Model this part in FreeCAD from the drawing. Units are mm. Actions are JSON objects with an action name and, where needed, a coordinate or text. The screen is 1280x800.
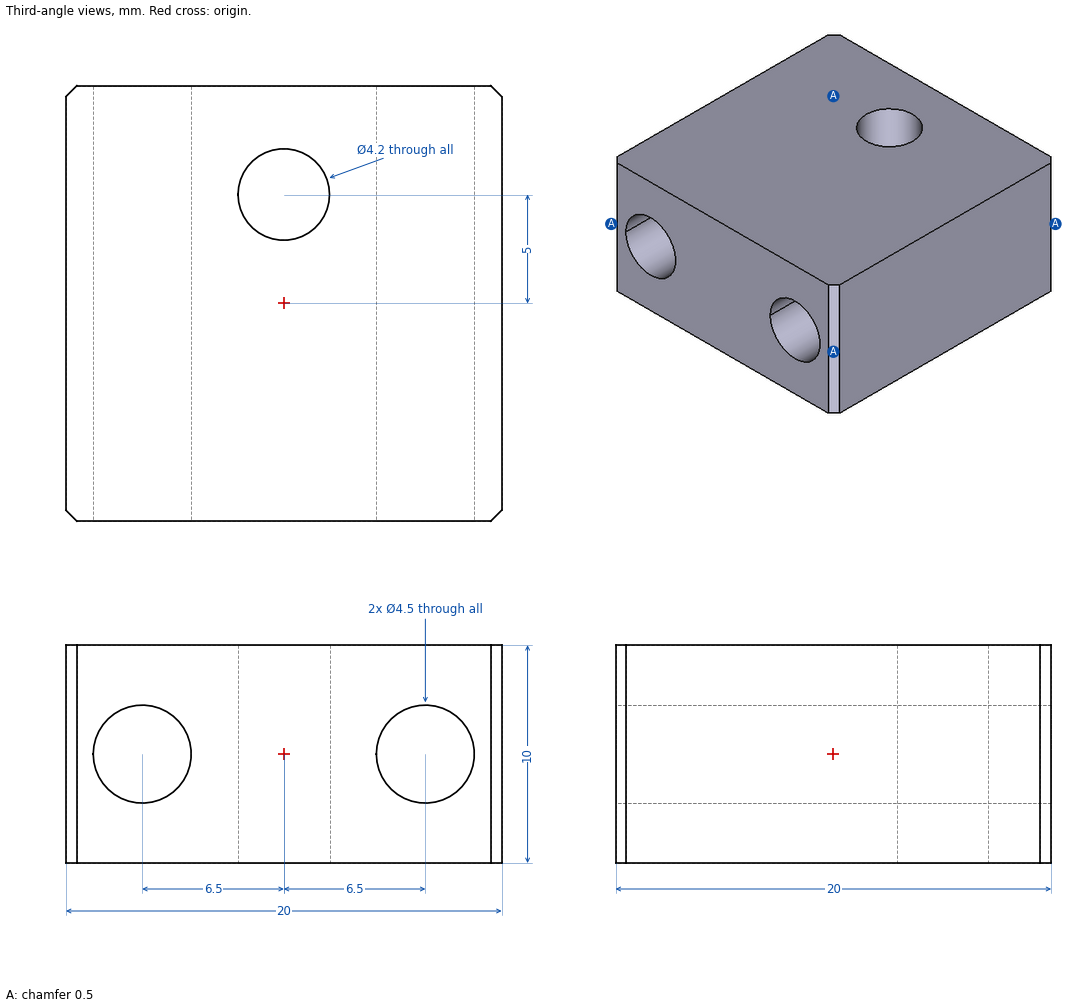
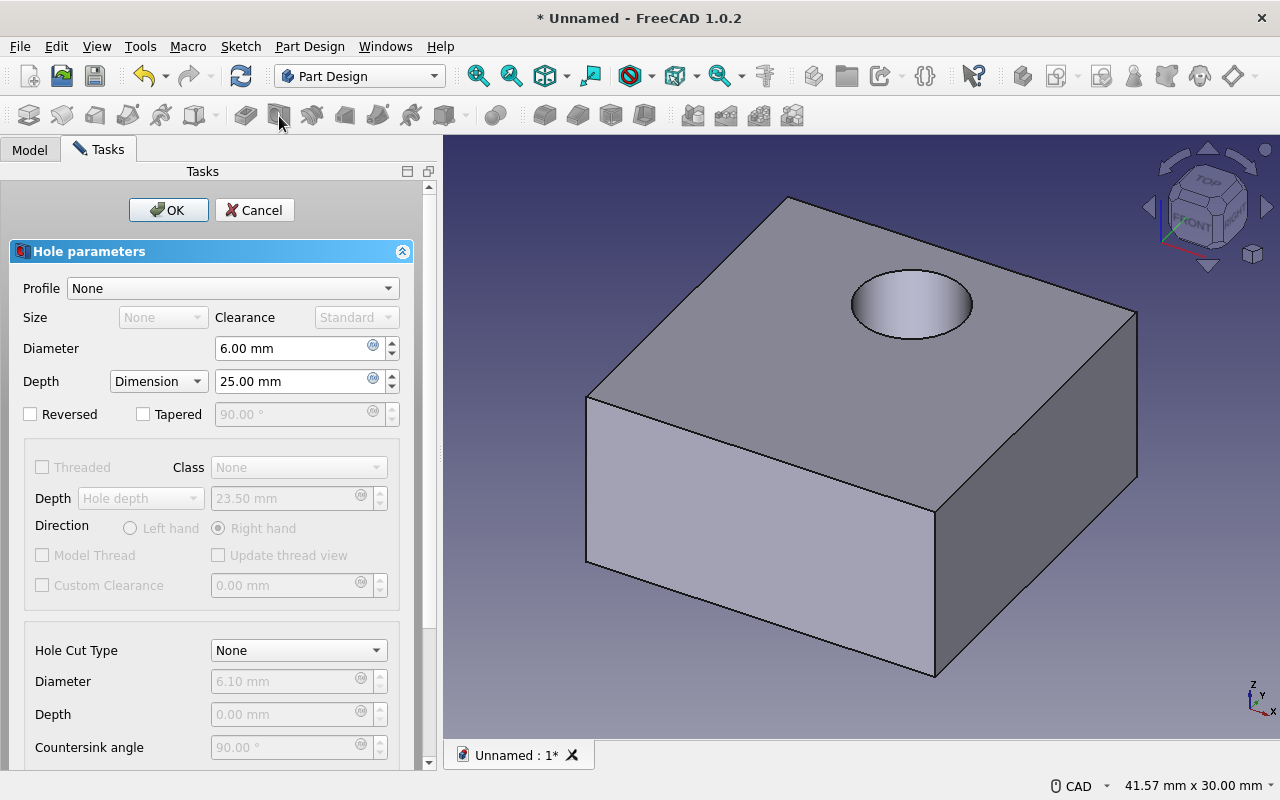
{"action": "triple_click", "coordinate": [300, 348]}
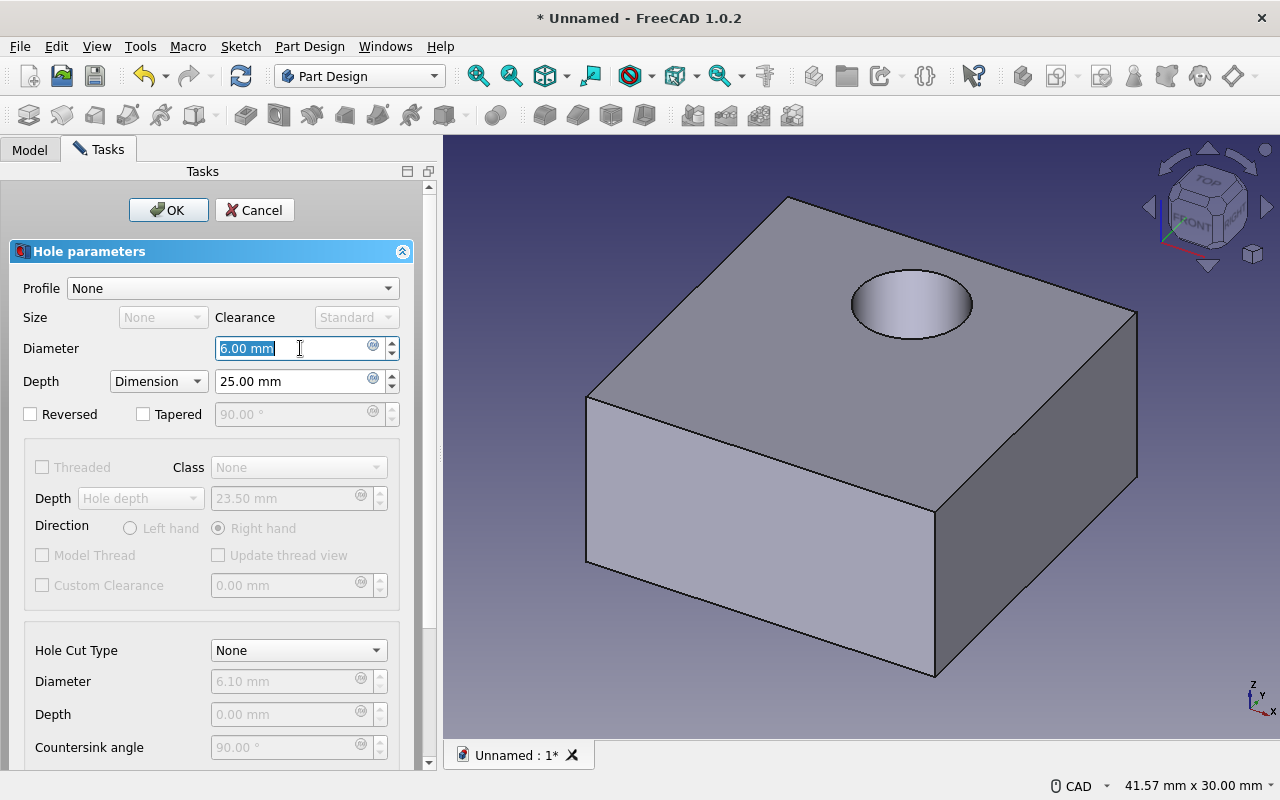
{"action": "type", "text": "4.2"}
{"action": "key", "text": "Tab"}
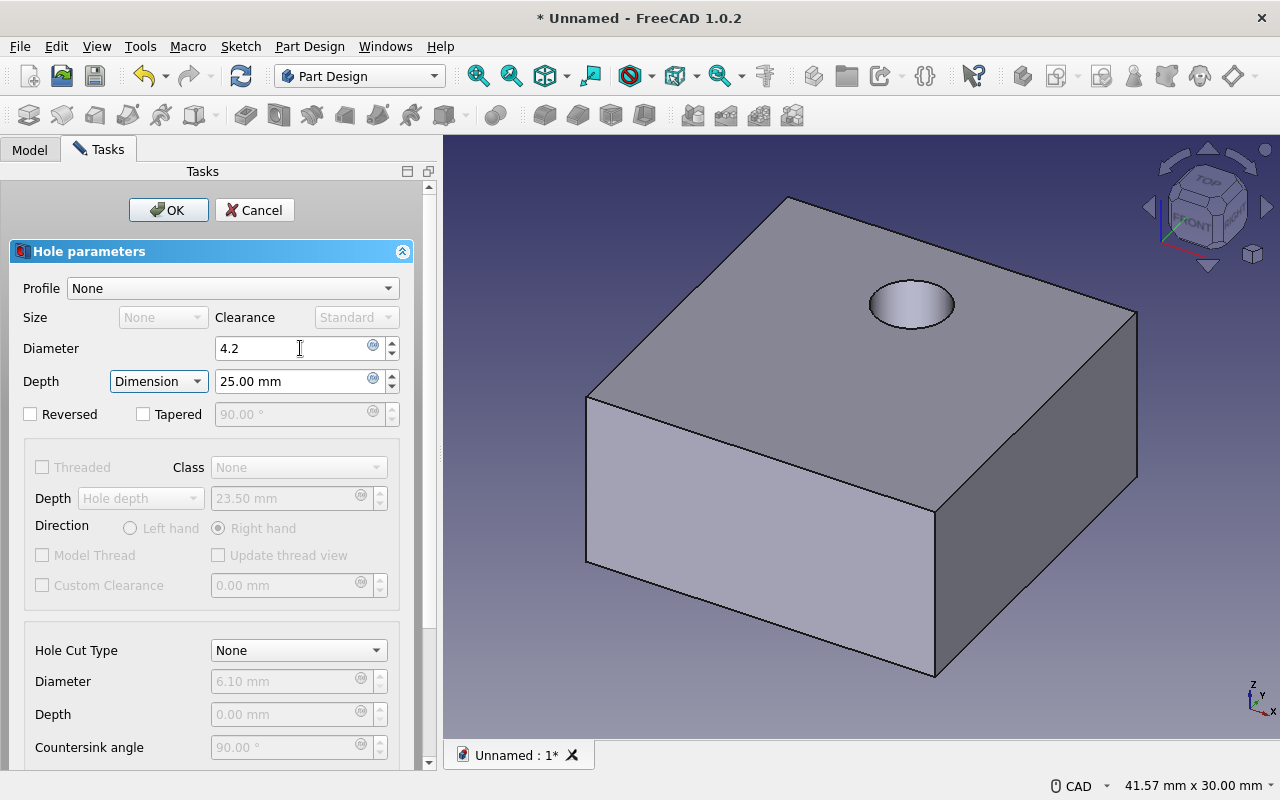
{"action": "left_click", "coordinate": [160, 382]}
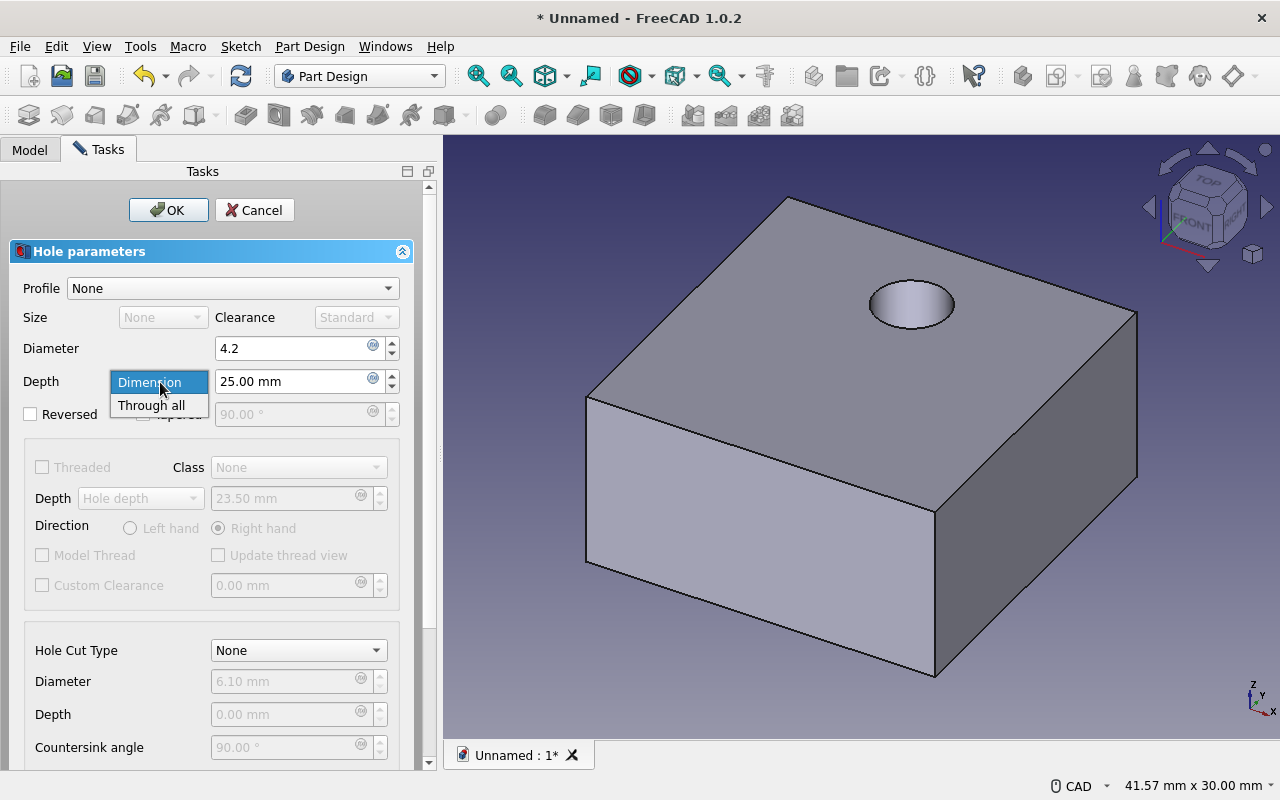
{"action": "left_click", "coordinate": [158, 406]}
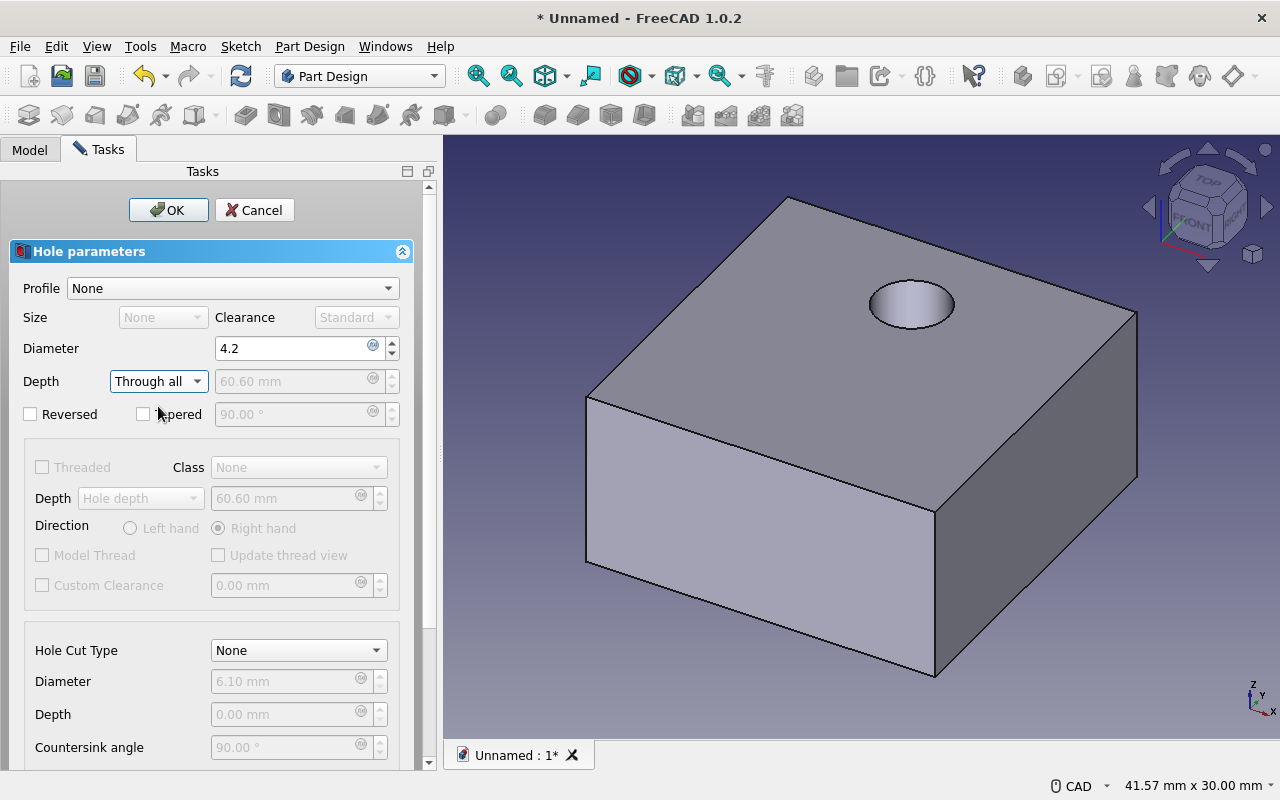
{"action": "left_click", "coordinate": [169, 210]}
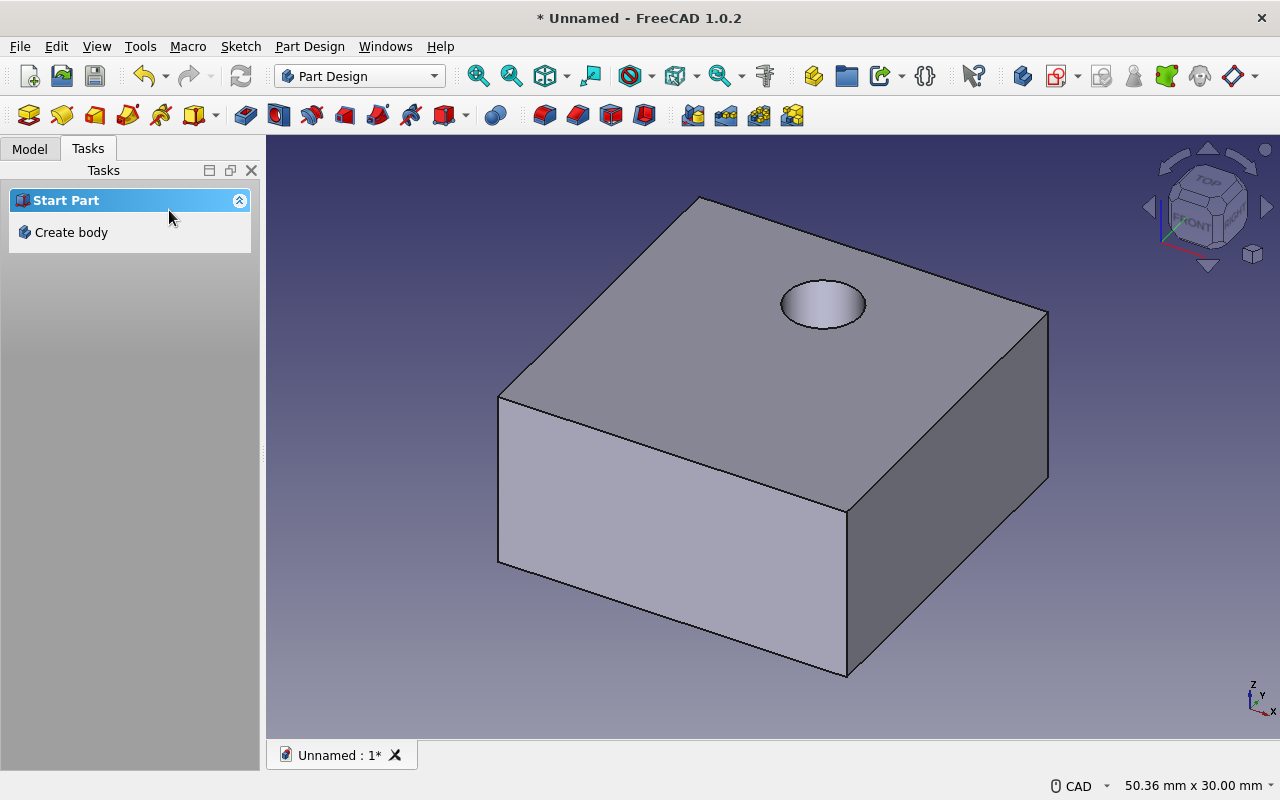
{"action": "key", "text": "4"}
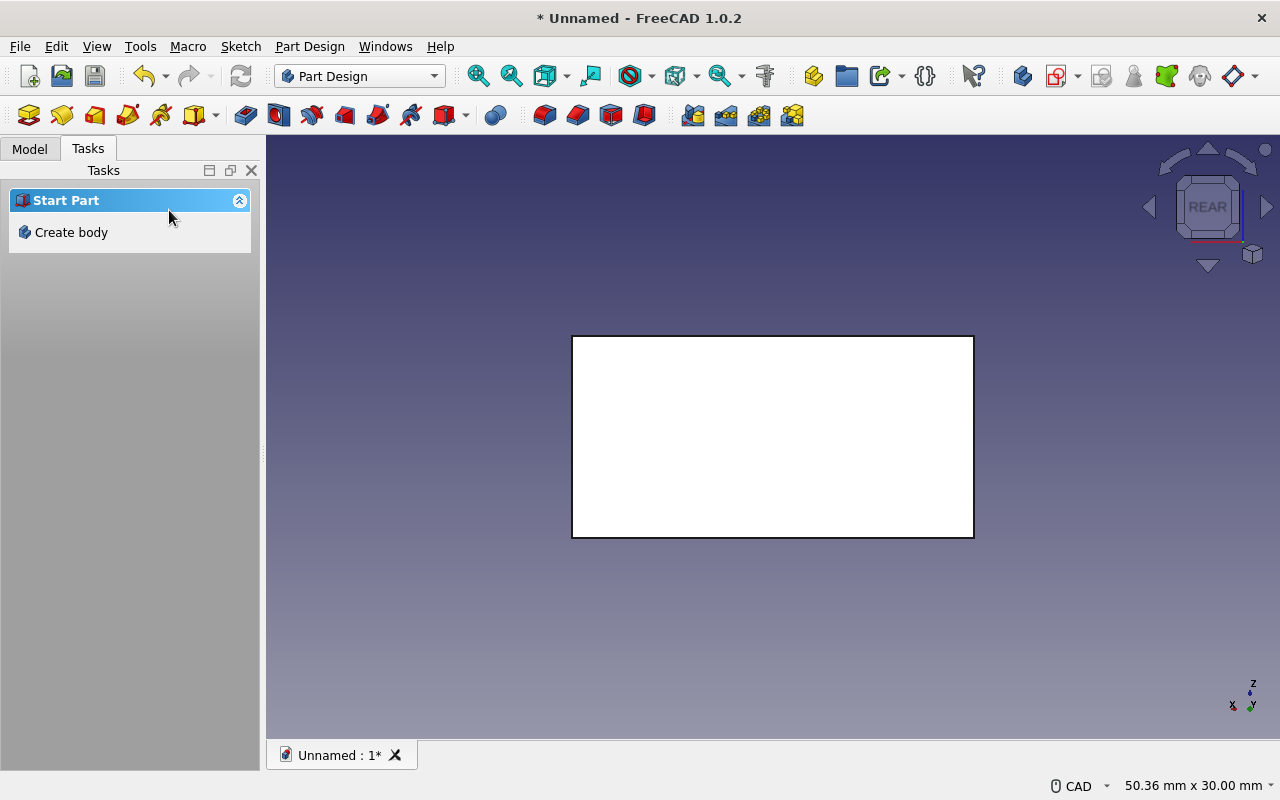
{"action": "key", "text": "v f"}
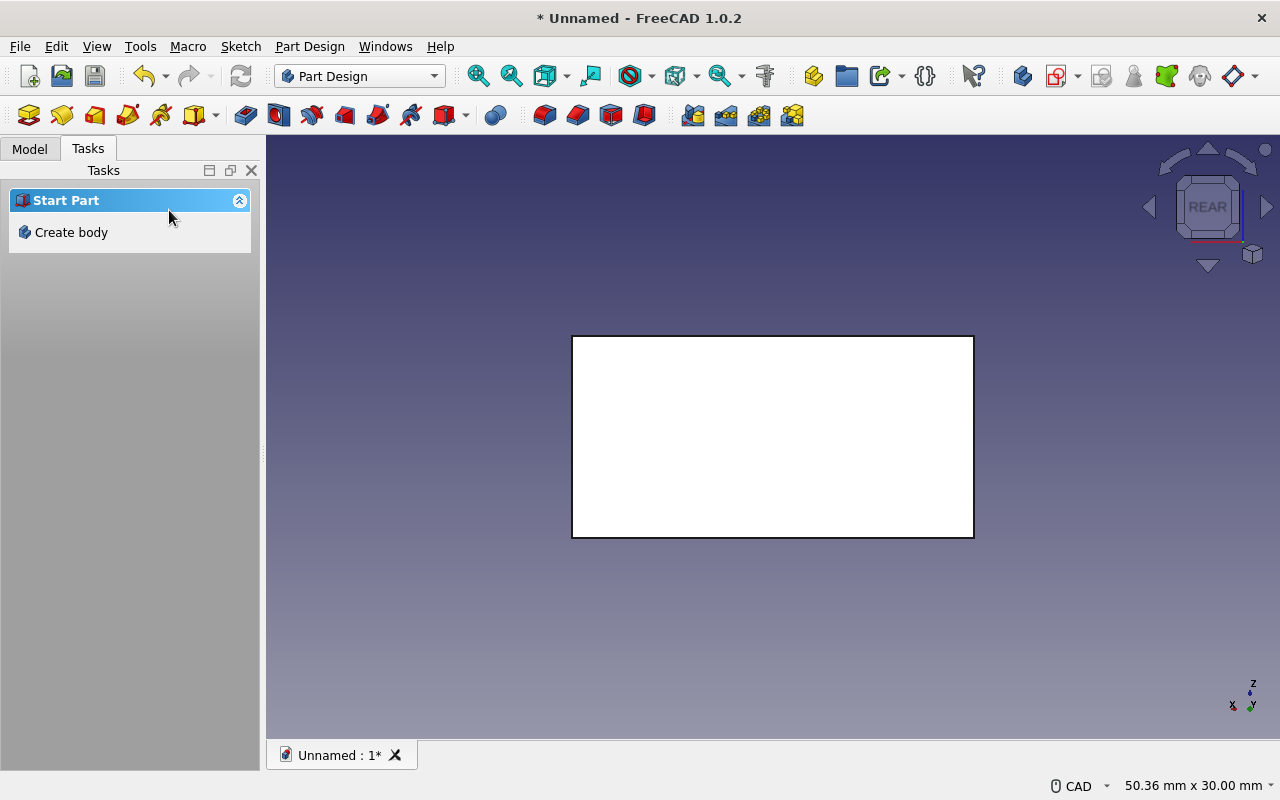
{"action": "left_click", "coordinate": [715, 436]}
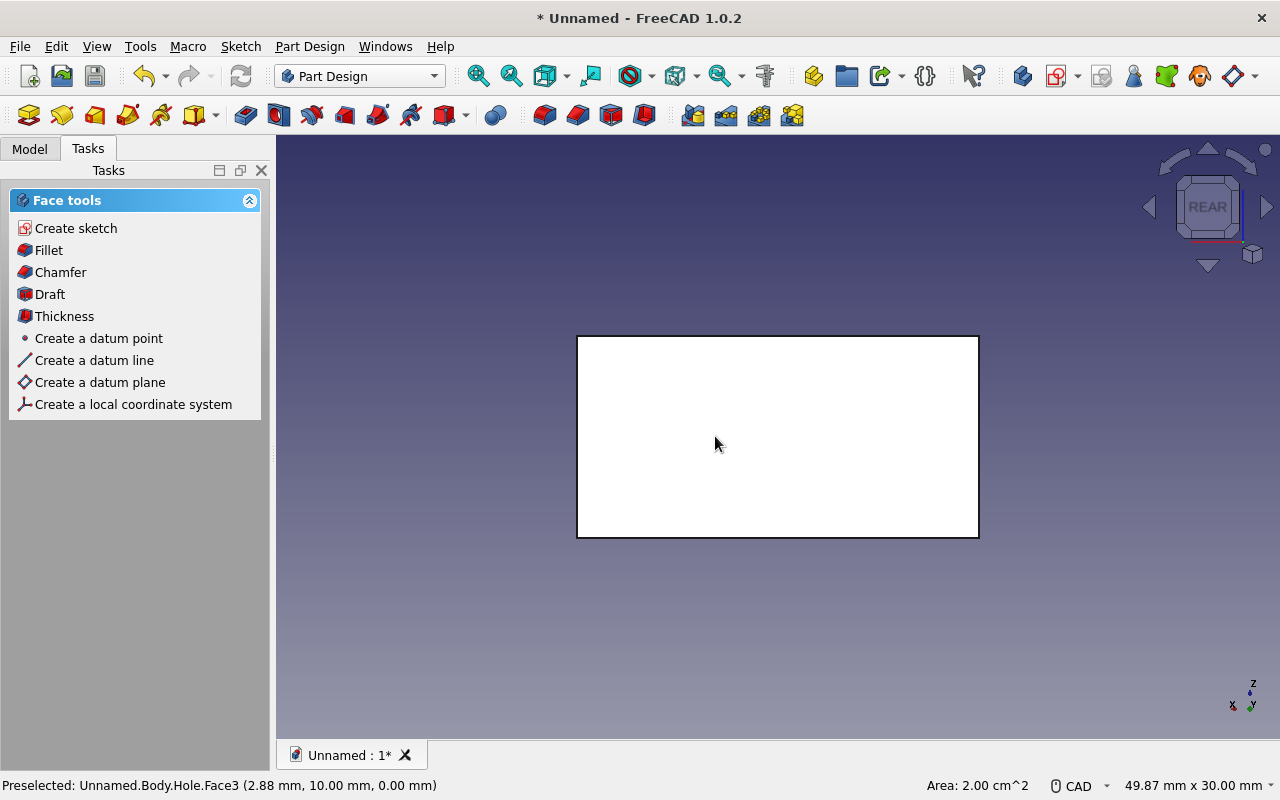
{"action": "left_click", "coordinate": [1056, 76]}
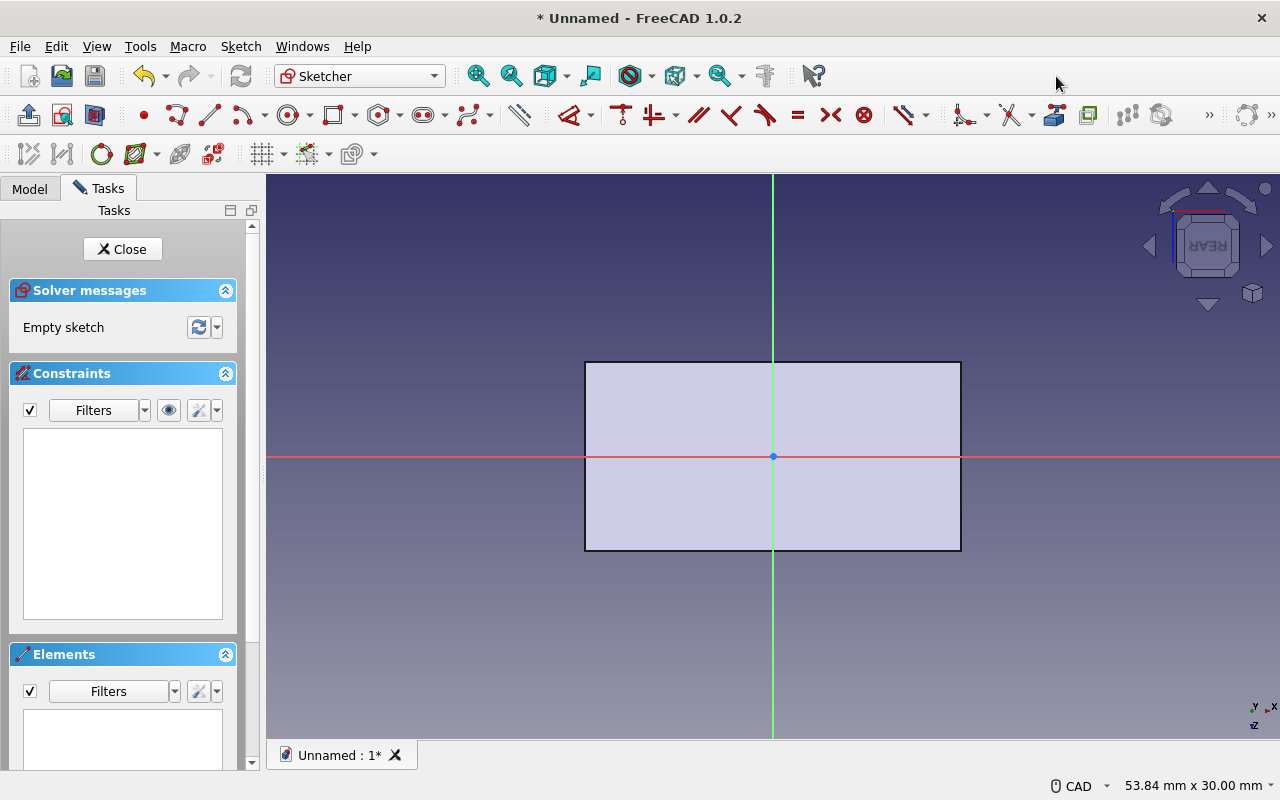
{"action": "scroll", "coordinate": [856, 456], "scroll_direction": "up", "scroll_amount": 3}